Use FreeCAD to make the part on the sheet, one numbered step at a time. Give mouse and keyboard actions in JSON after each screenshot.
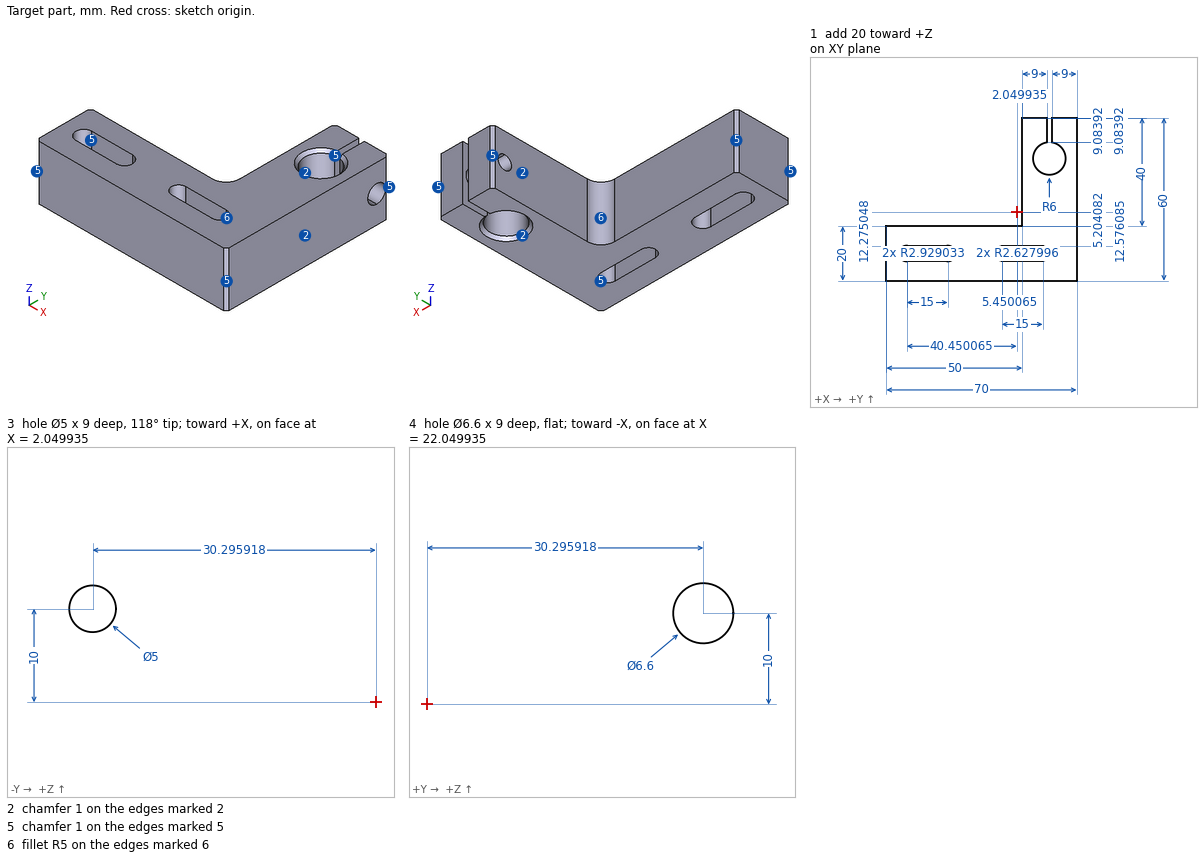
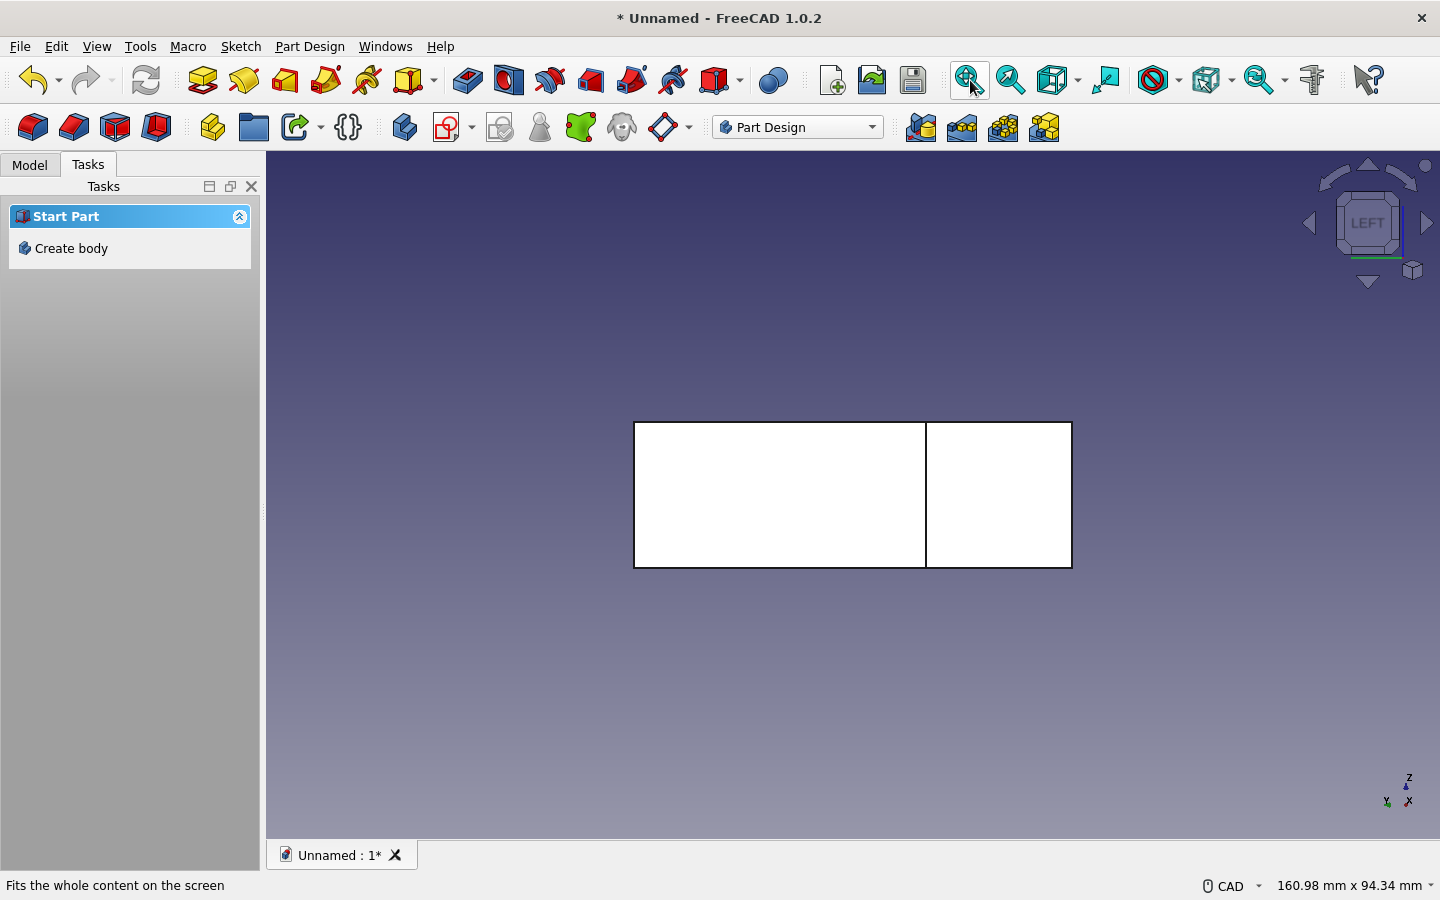
{"action": "left_click", "coordinate": [738, 494]}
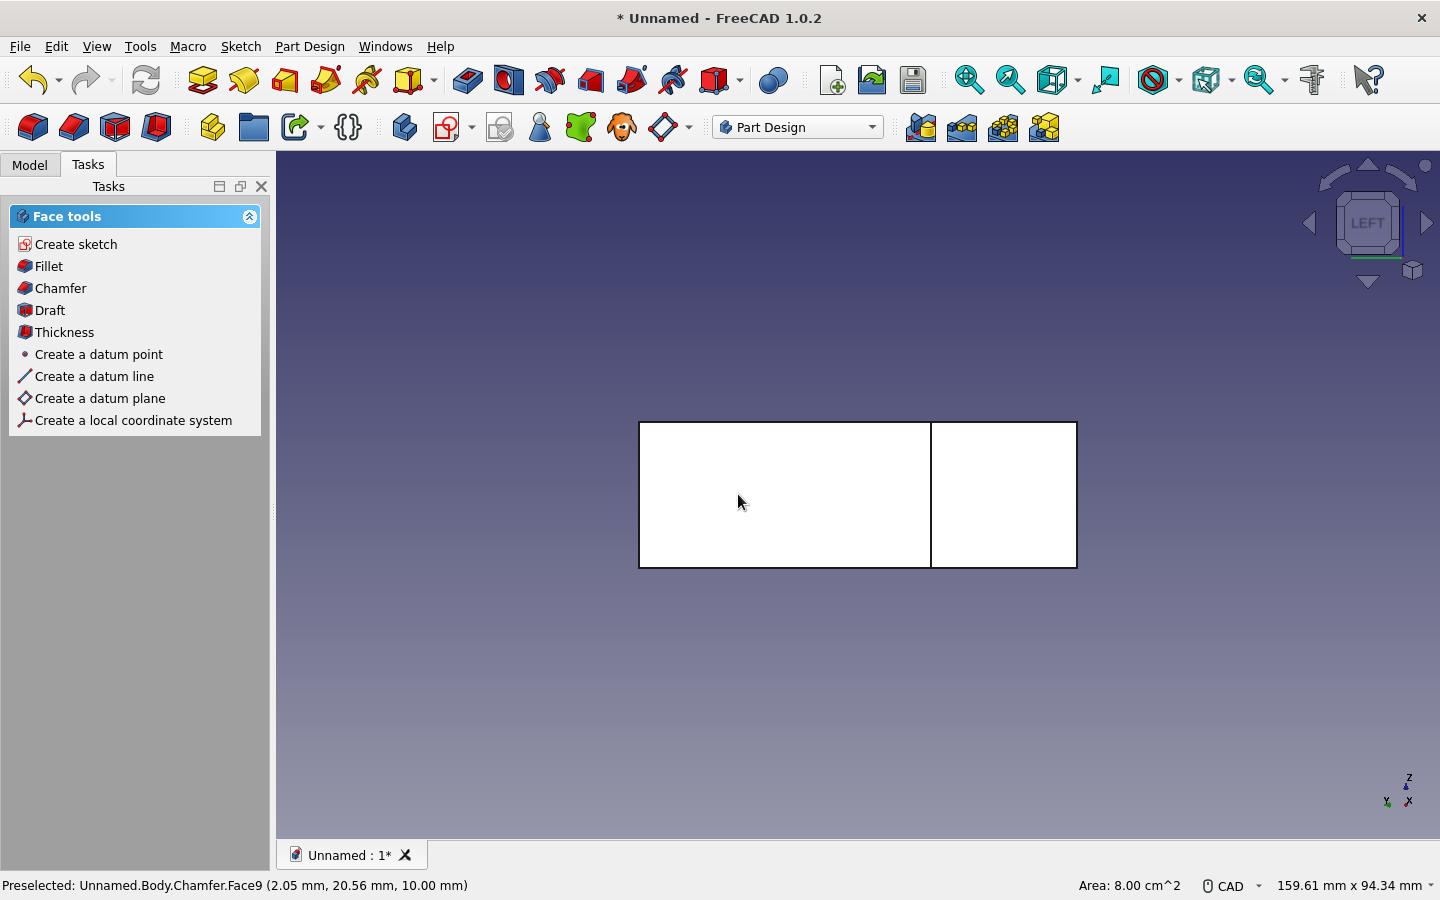
{"action": "left_click", "coordinate": [446, 128]}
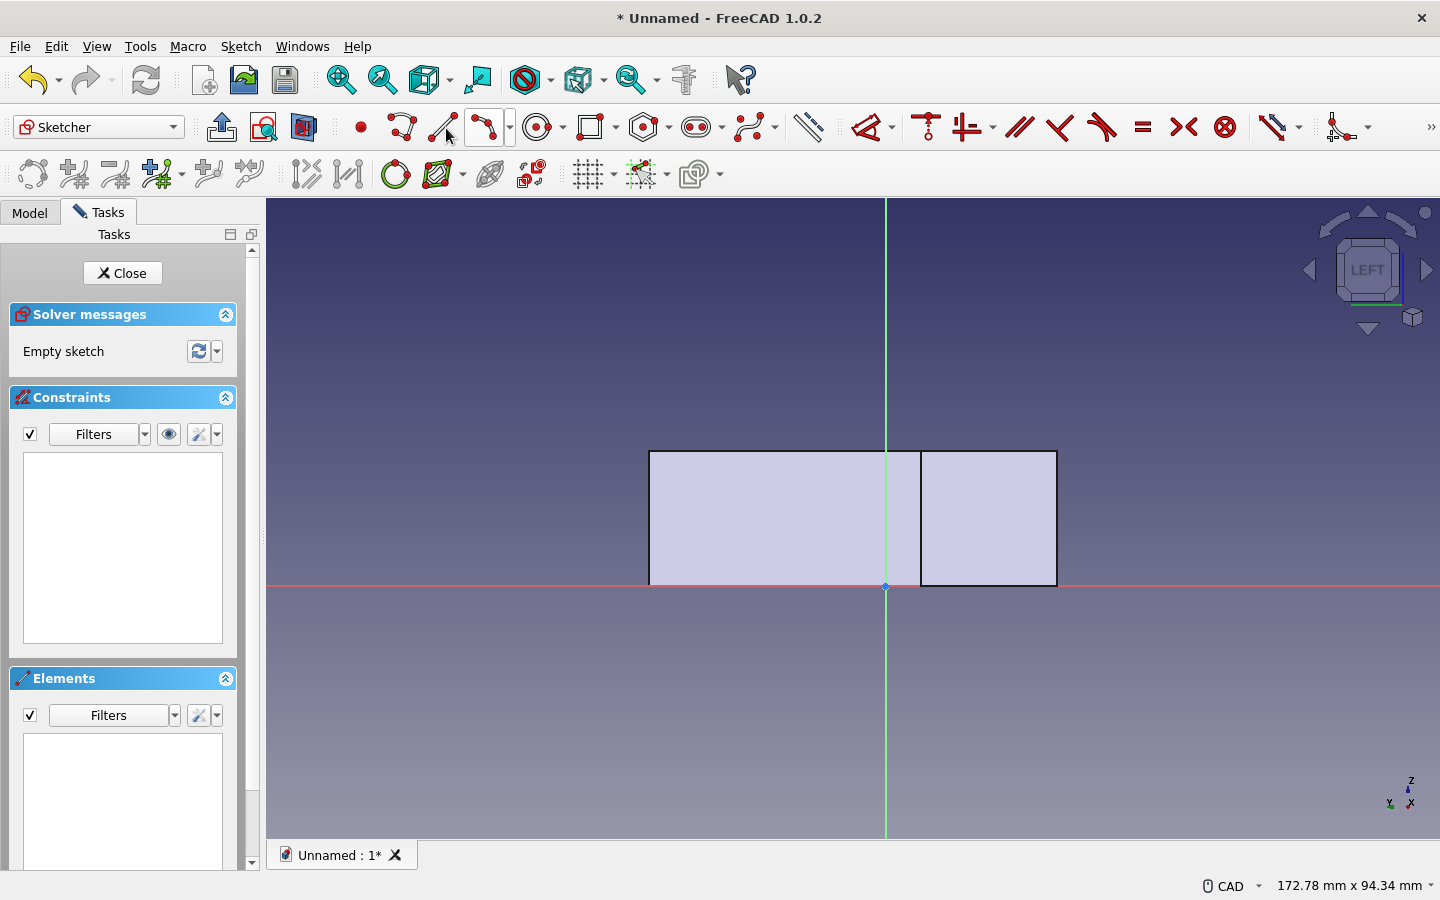
{"action": "left_click", "coordinate": [304, 128]}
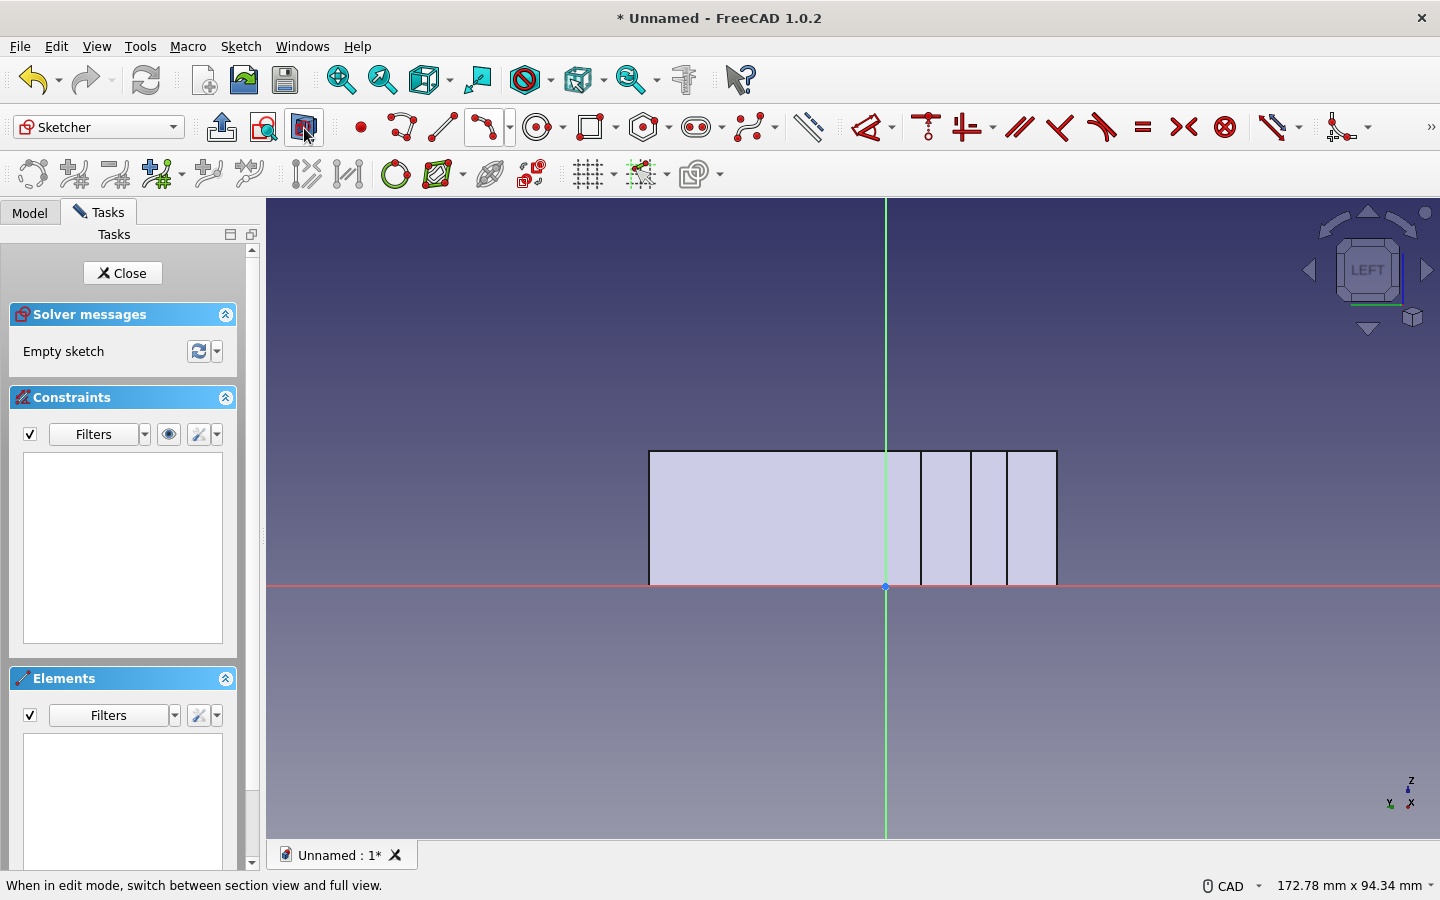
{"action": "scroll", "coordinate": [669, 518], "scroll_direction": "up", "scroll_amount": 12}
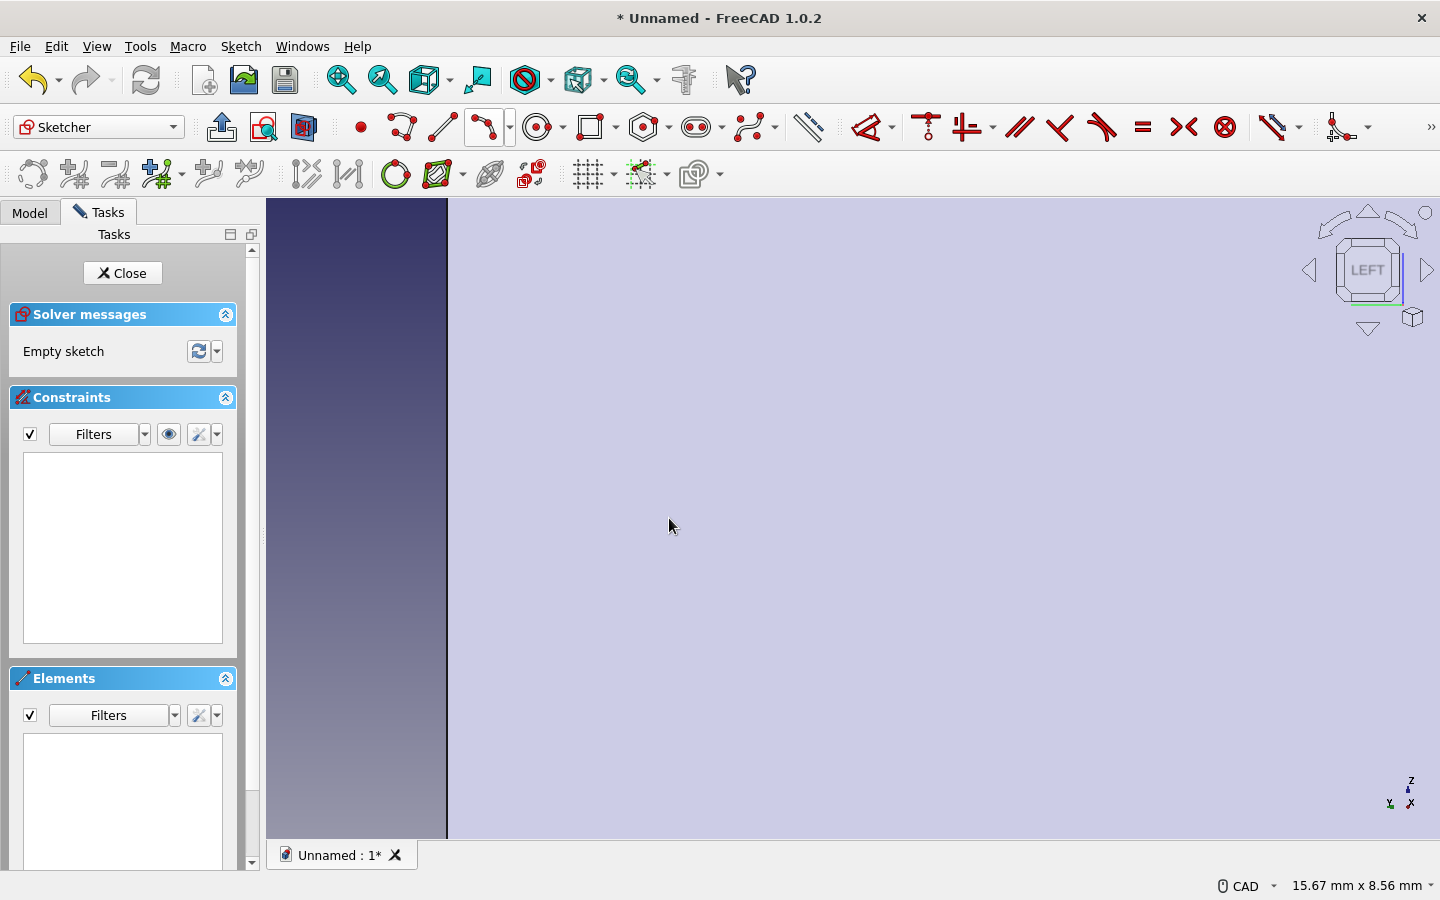
{"action": "left_click", "coordinate": [536, 128]}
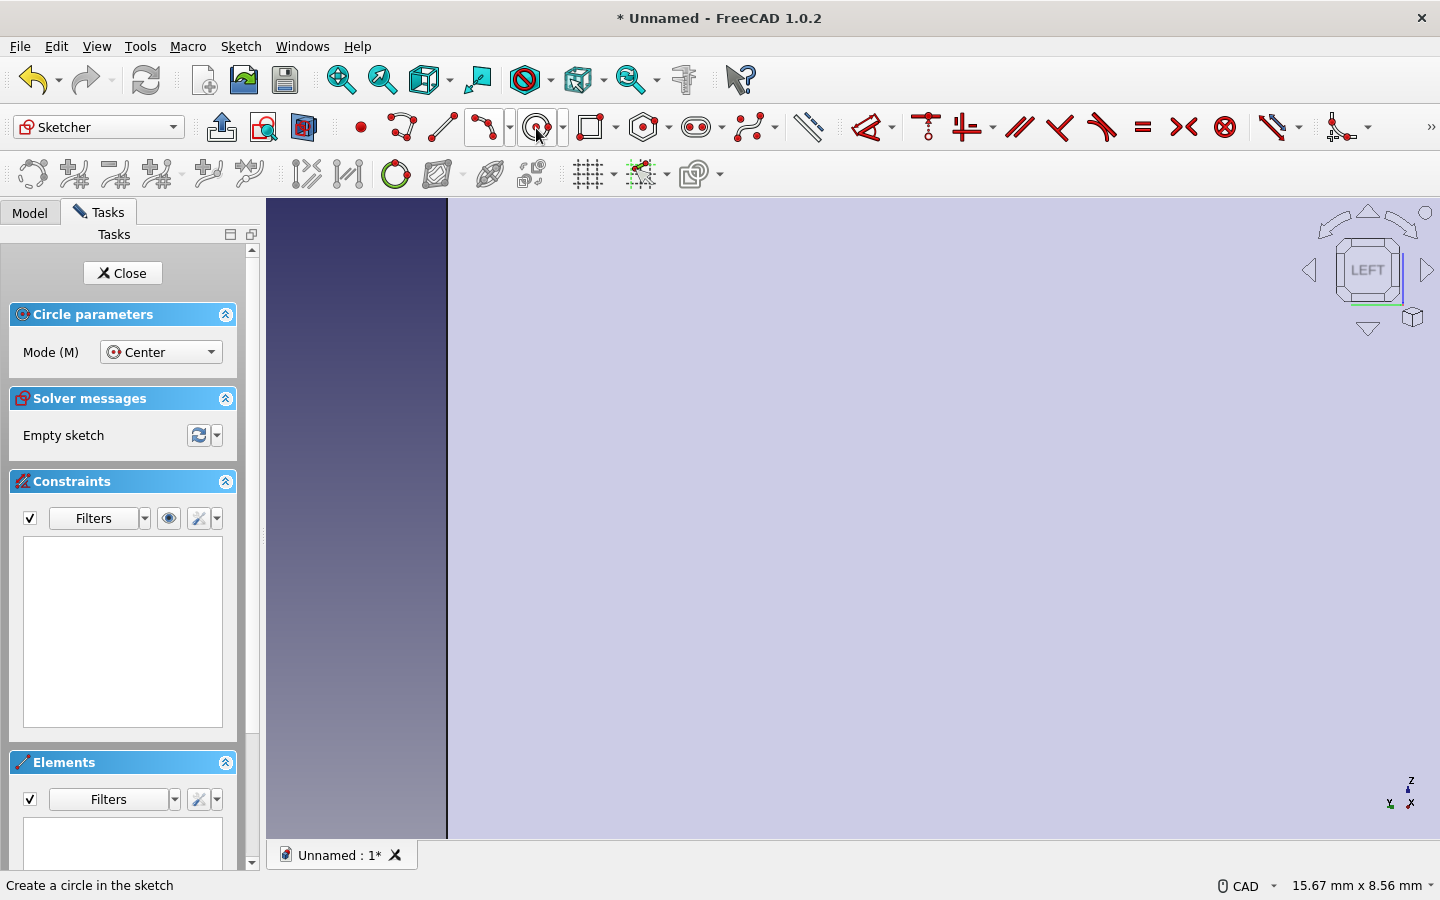
{"action": "left_click", "coordinate": [784, 519]}
{"action": "left_click", "coordinate": [916, 386]}
{"action": "key", "text": "Escape"}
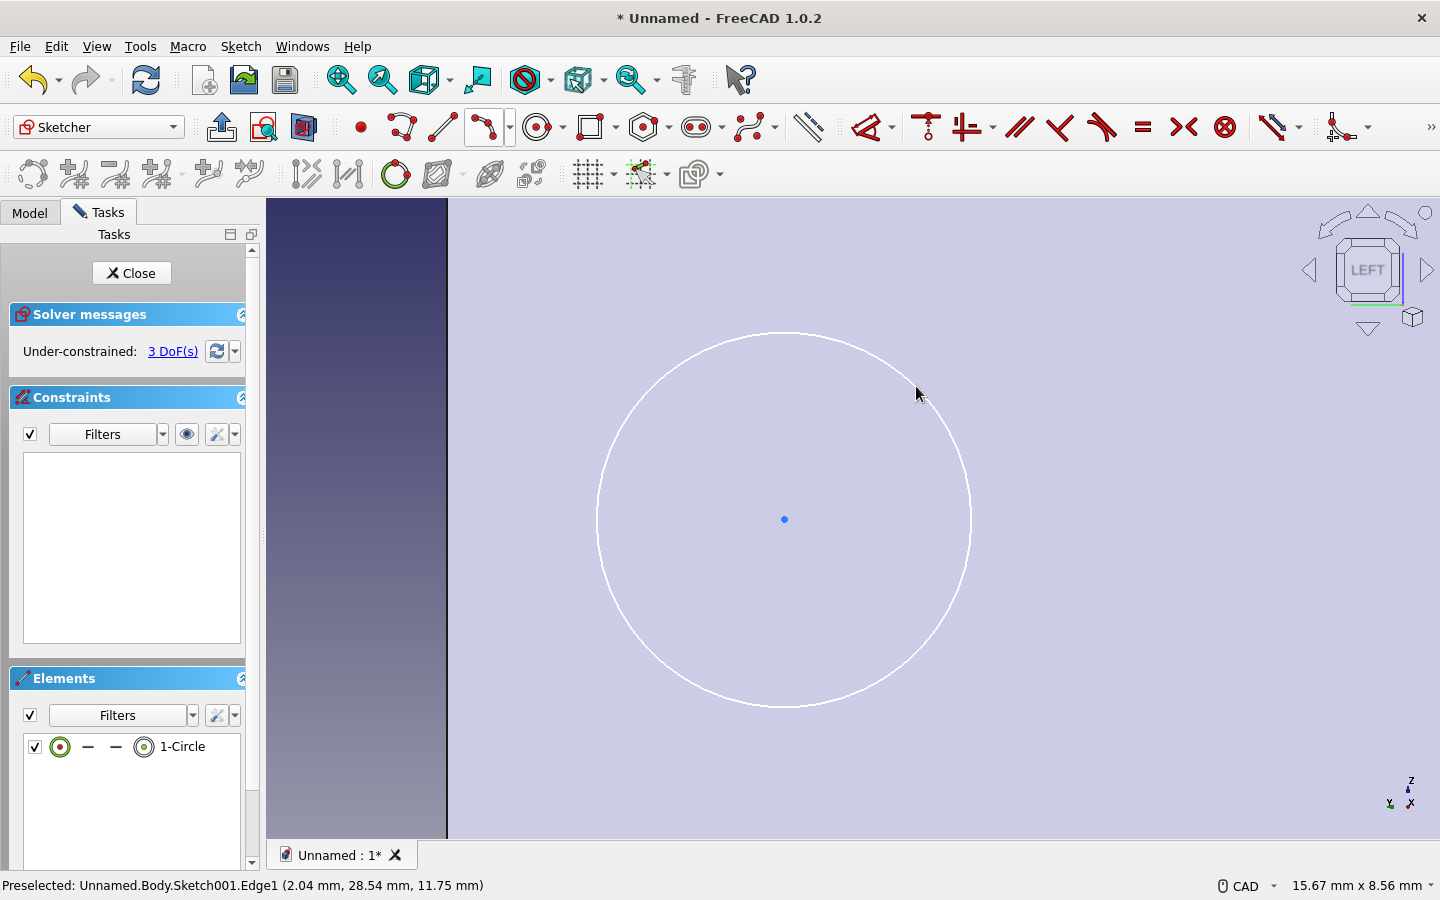
{"action": "left_click", "coordinate": [866, 128]}